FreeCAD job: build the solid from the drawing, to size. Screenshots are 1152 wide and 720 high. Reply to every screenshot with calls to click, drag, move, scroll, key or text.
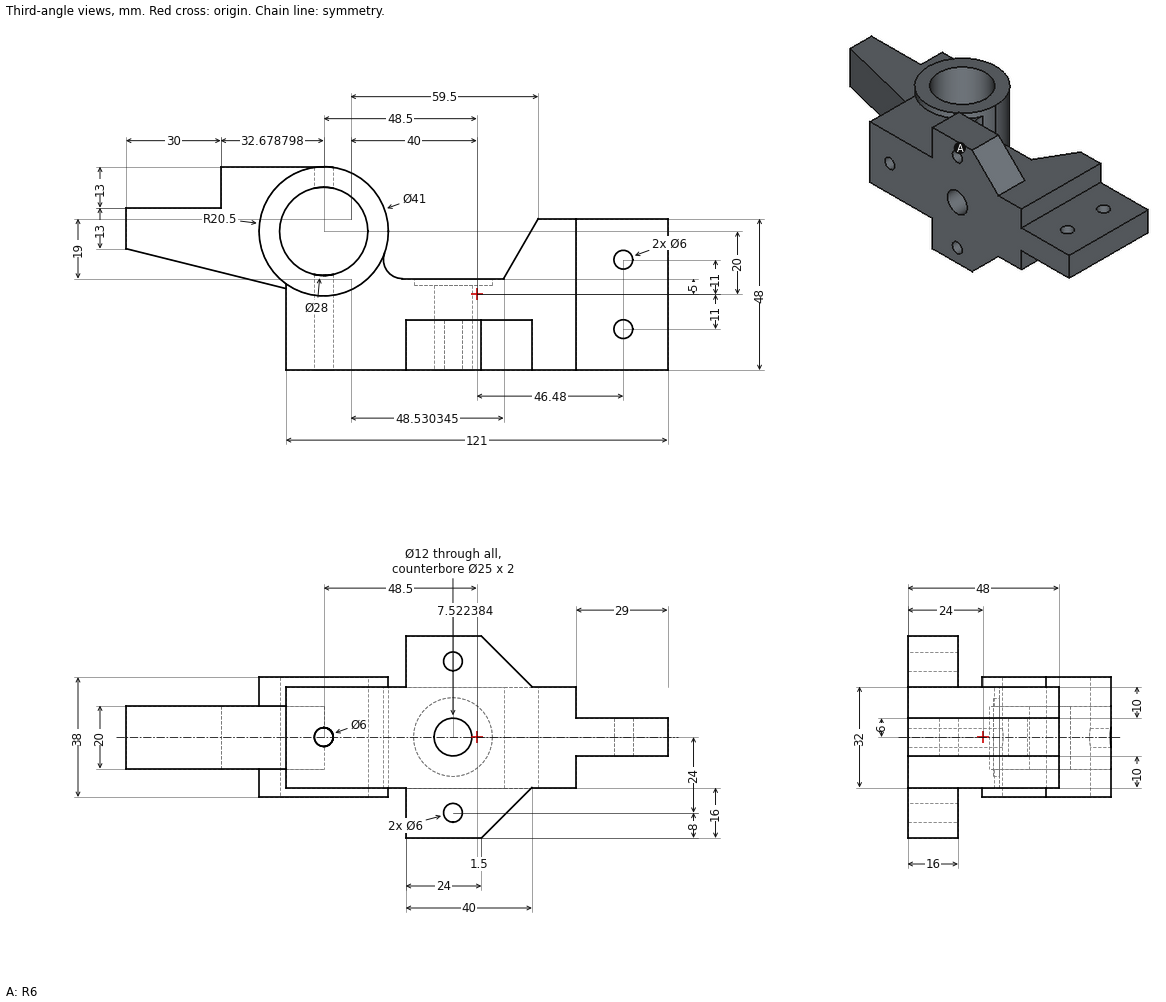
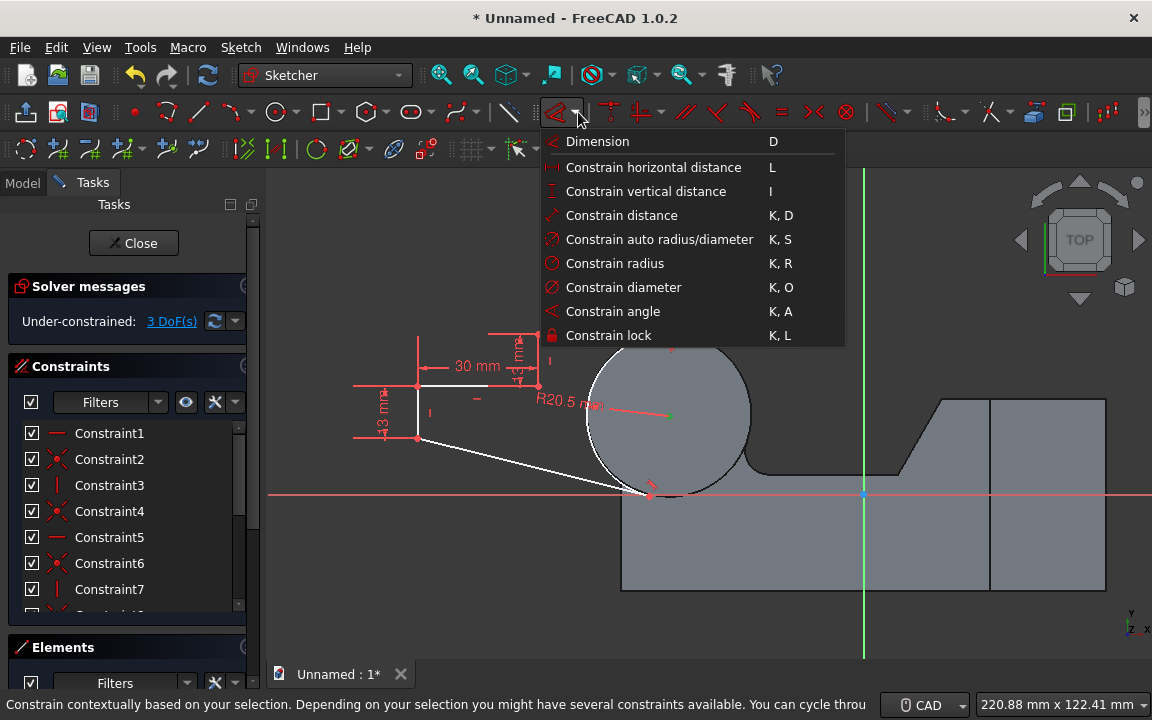
click(693, 191)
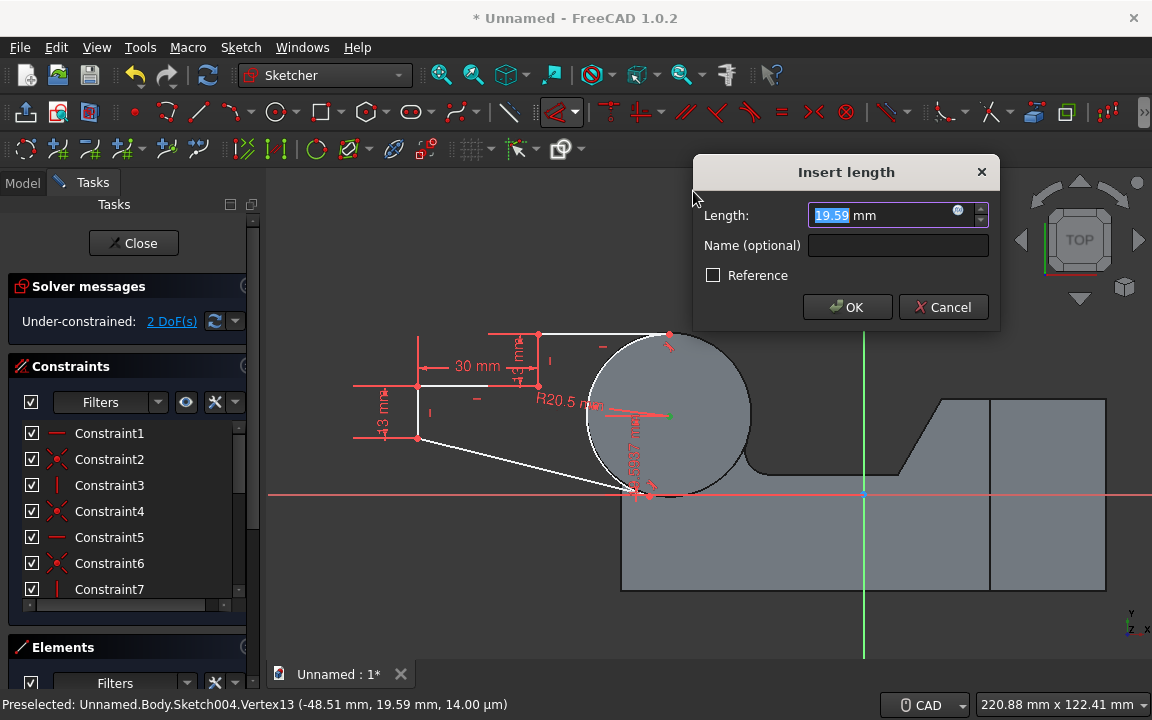
text(20)
key(Return)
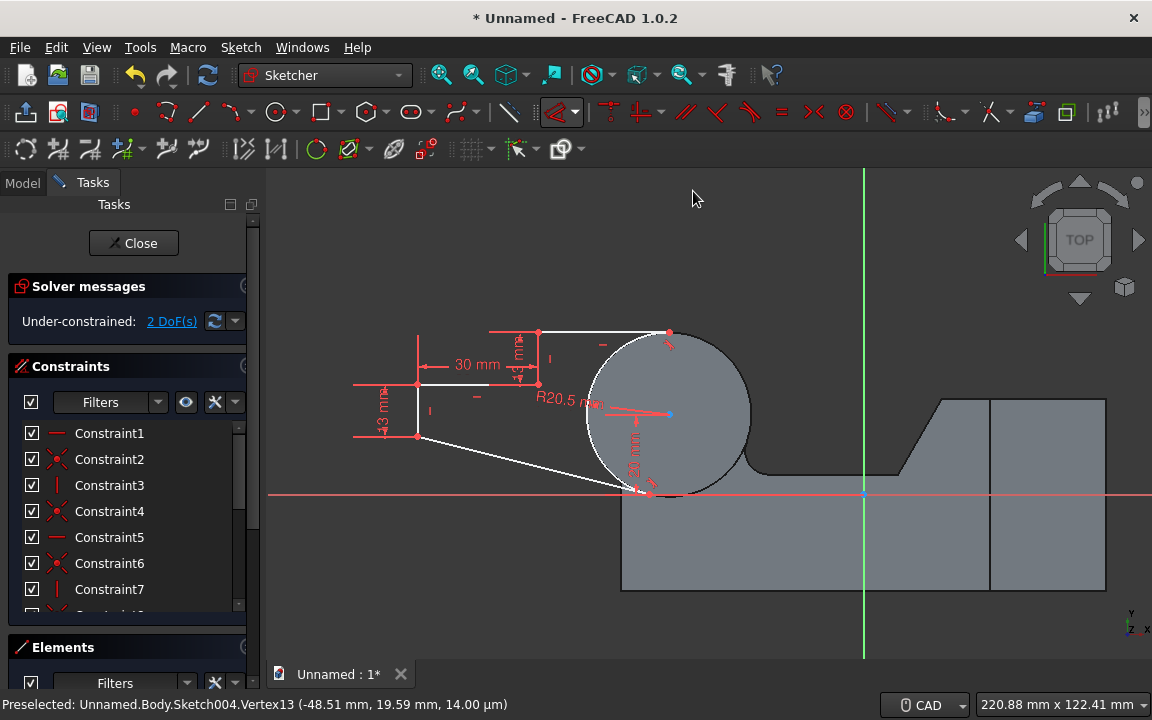
click(669, 332)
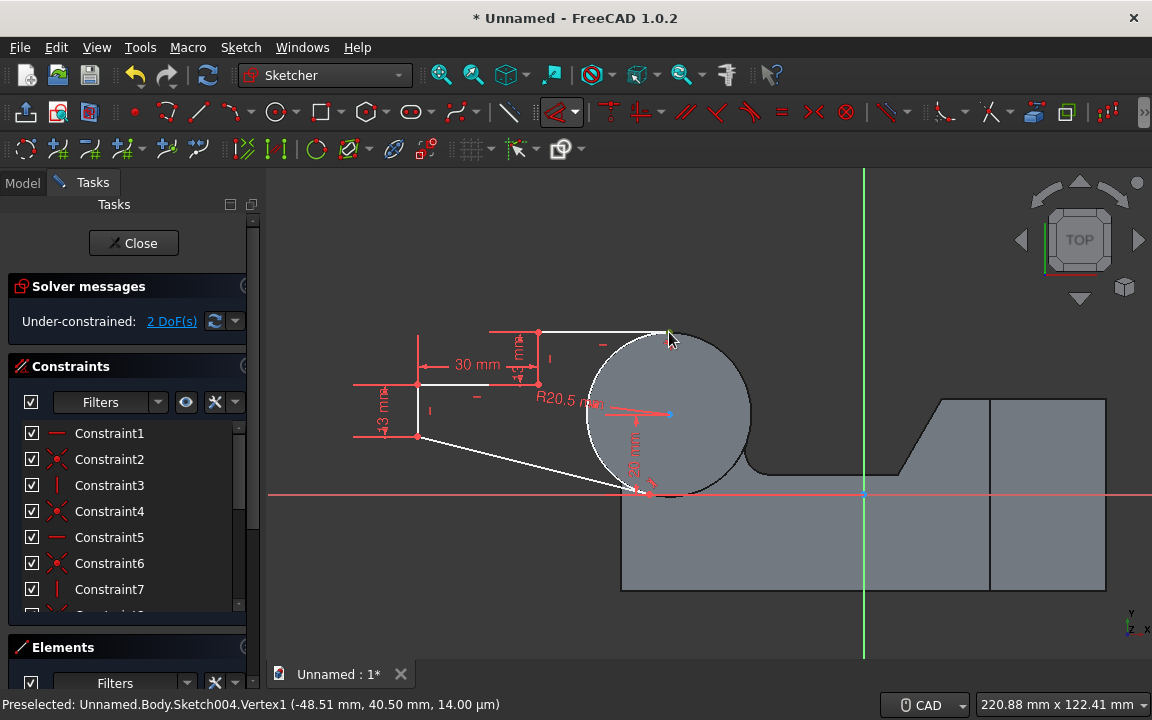
key(l)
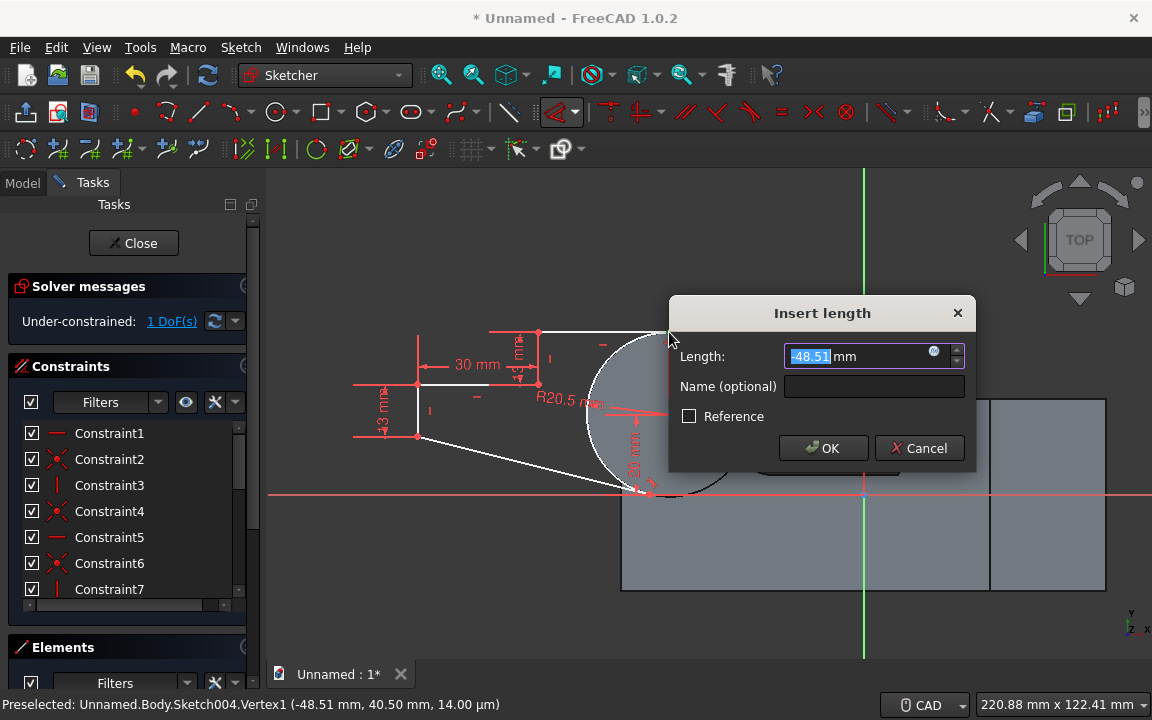
text(-48.5)
key(Return)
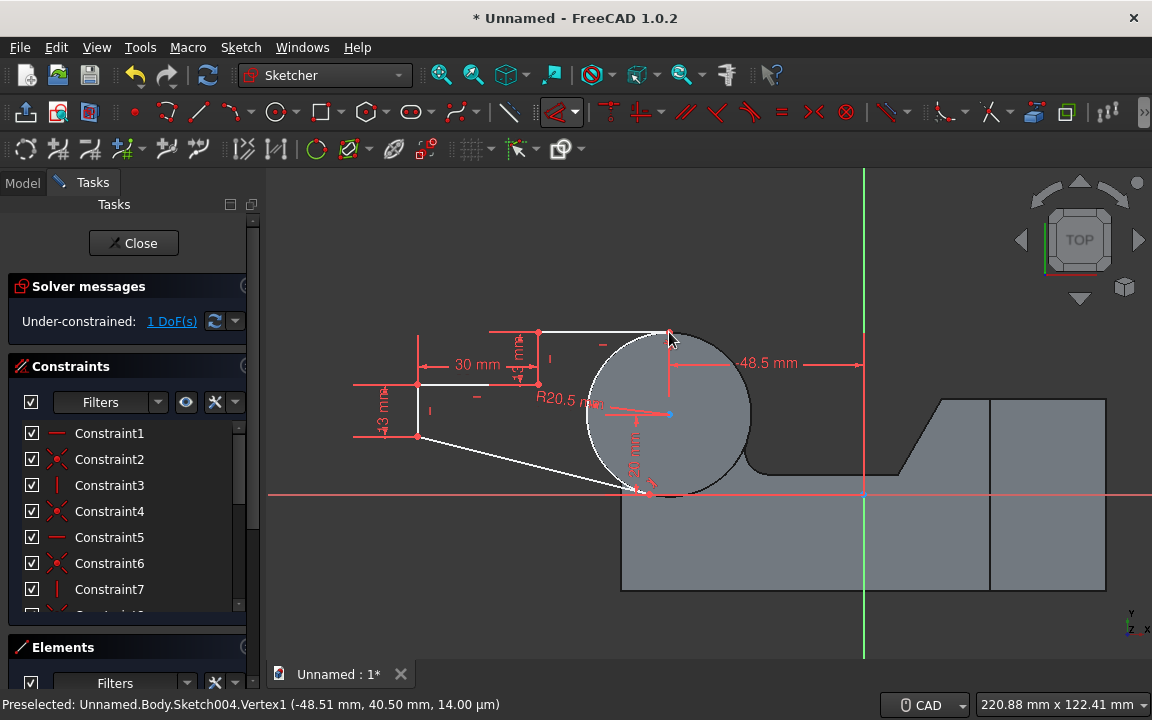
click(577, 332)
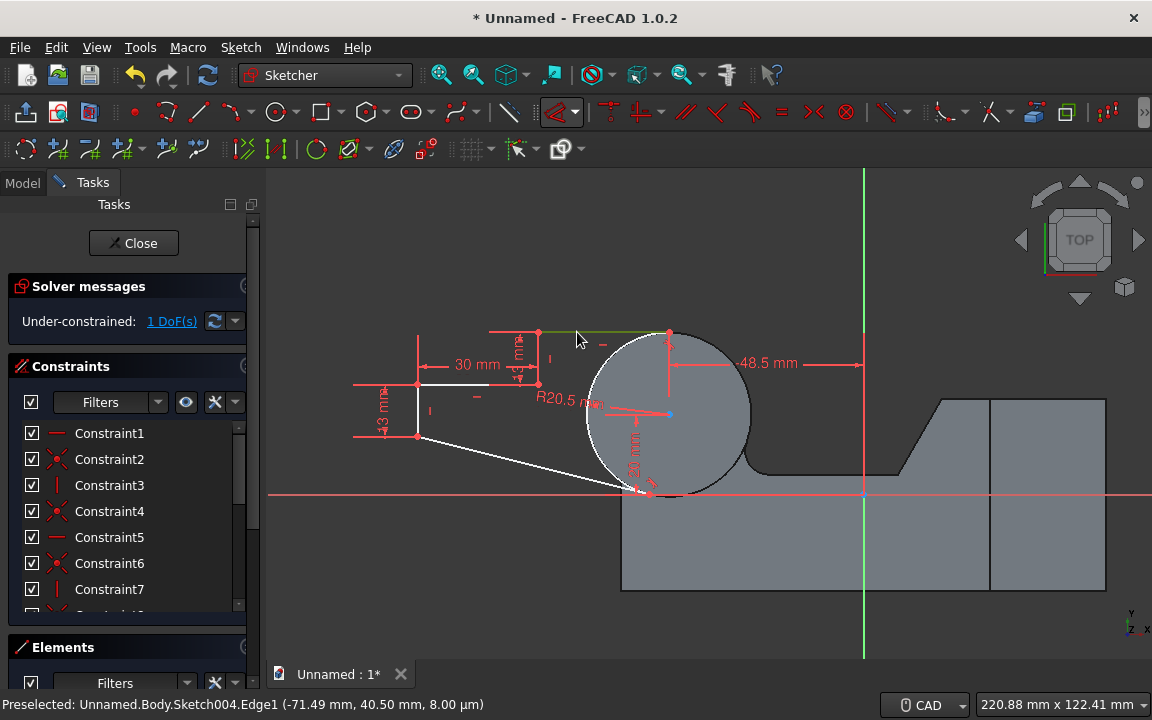
key(l)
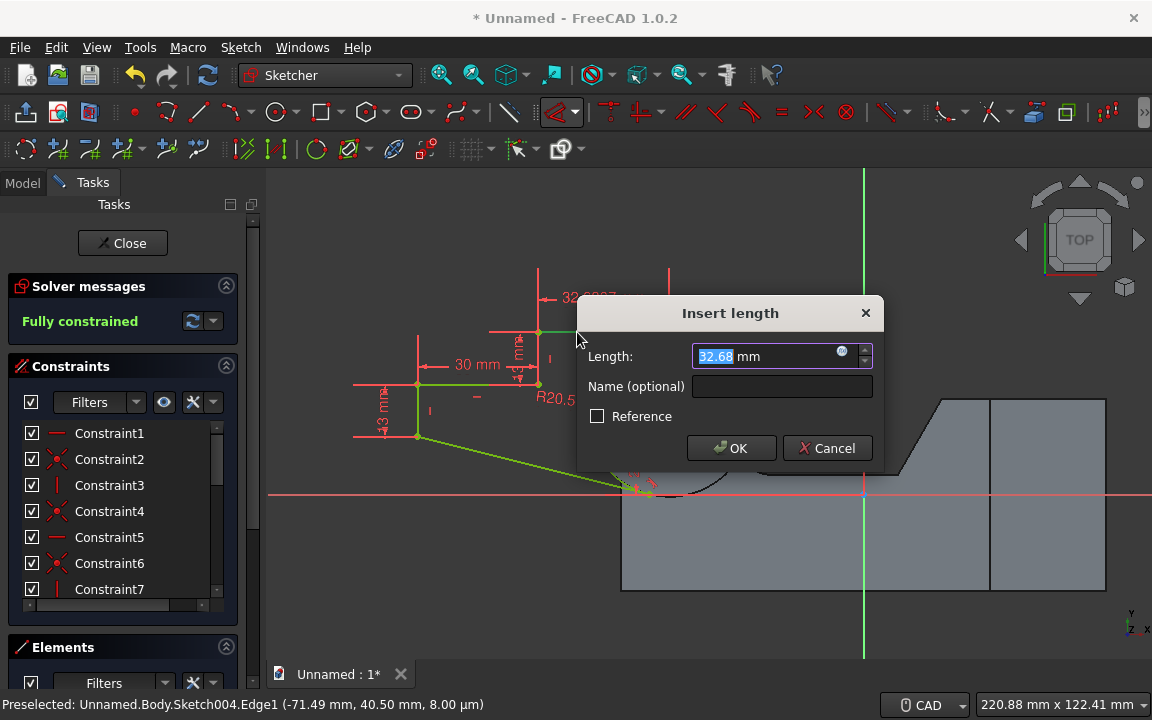
text(32.678798)
key(Return)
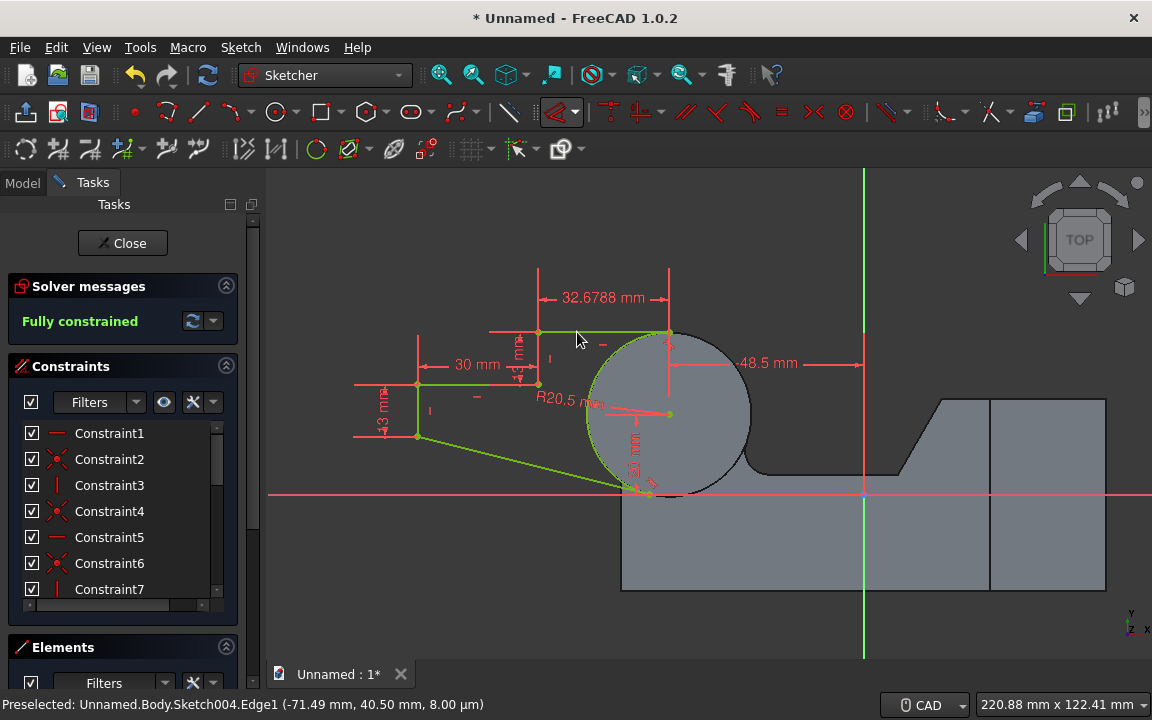
click(123, 243)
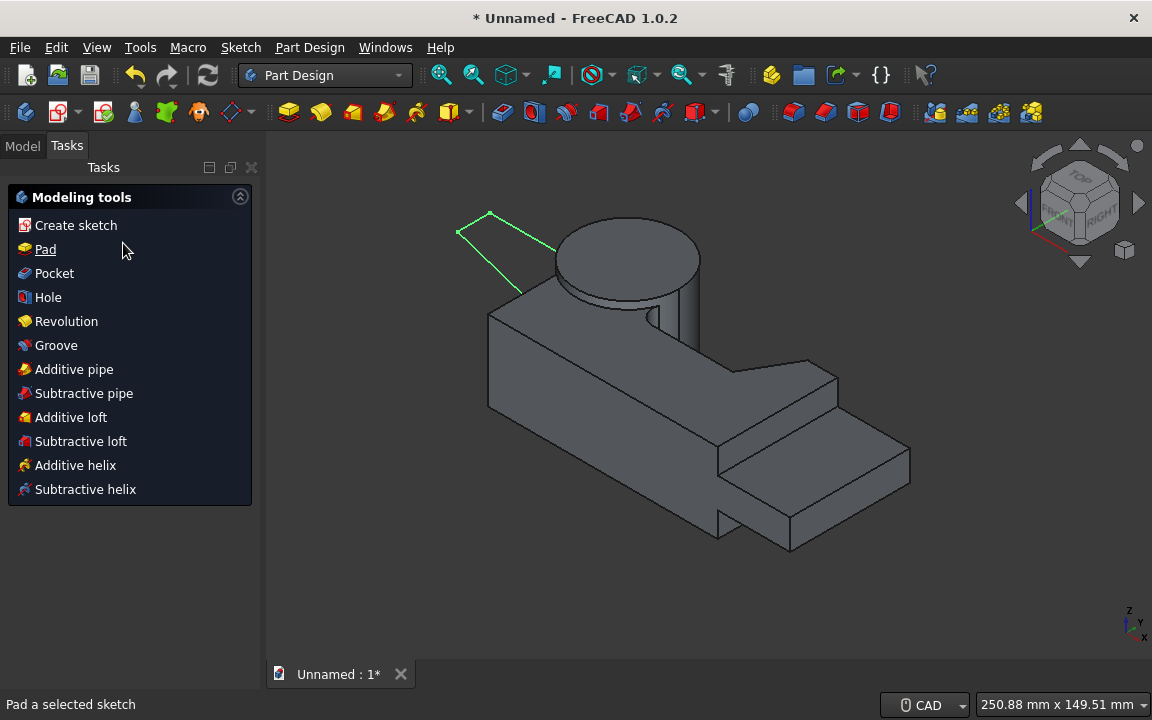
click(290, 112)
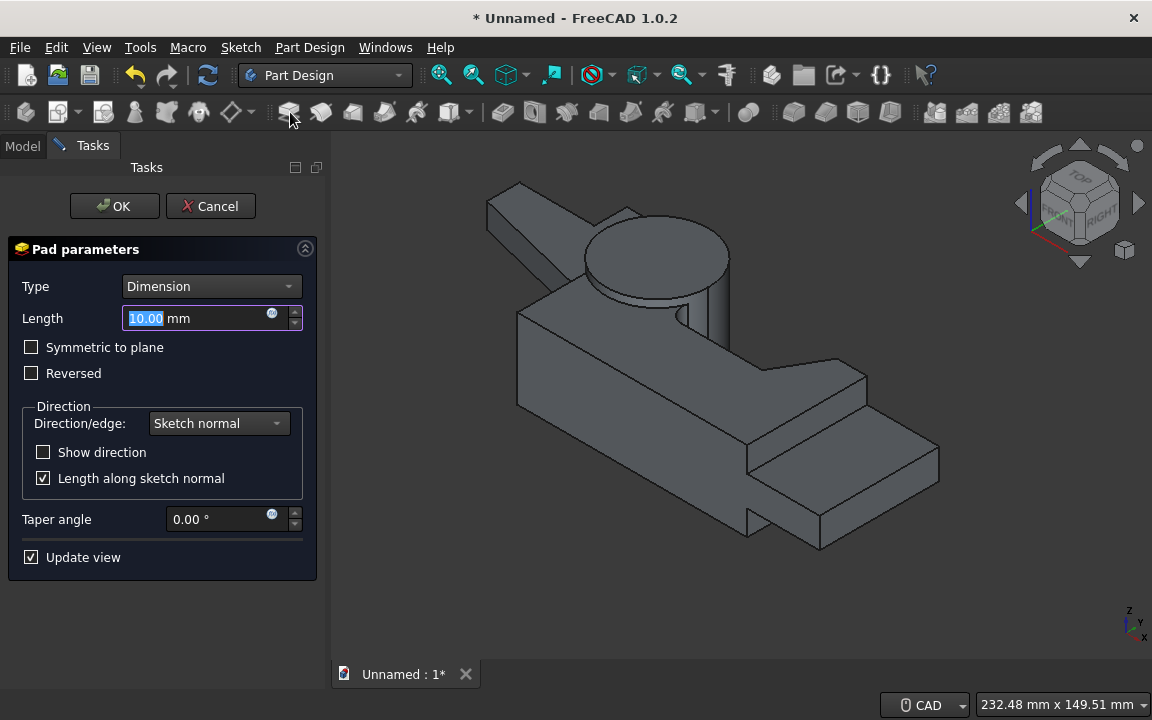
text(20)
key(Tab)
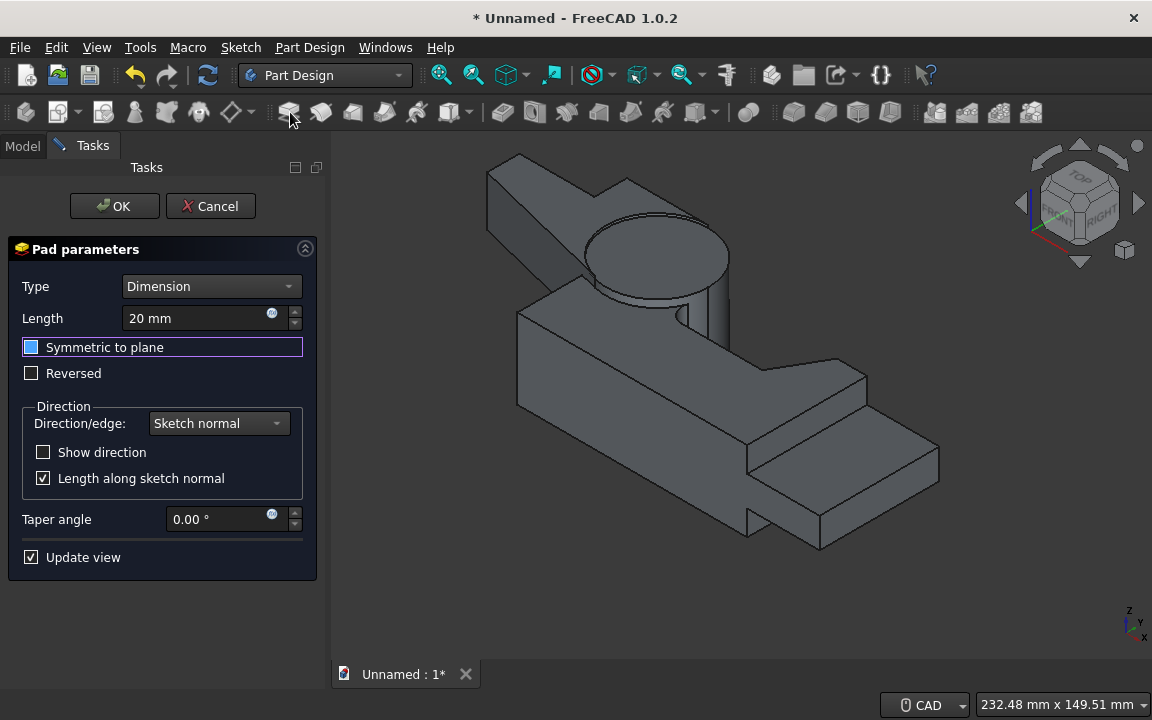
click(30, 347)